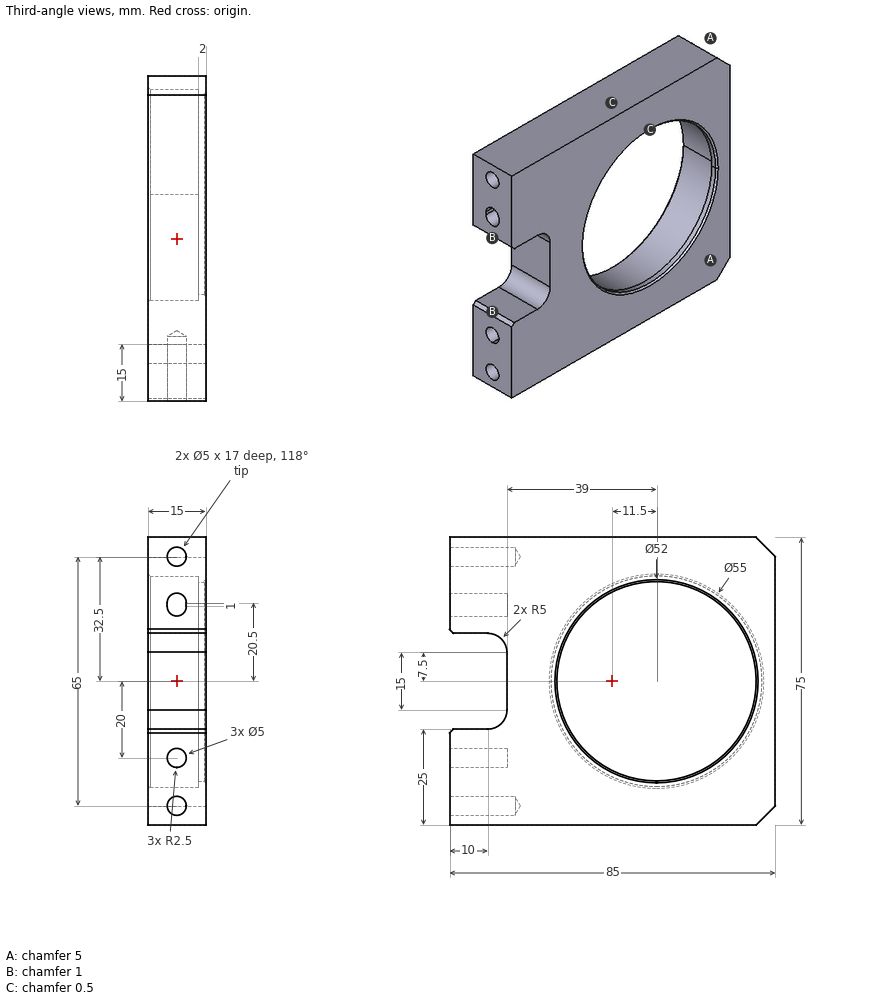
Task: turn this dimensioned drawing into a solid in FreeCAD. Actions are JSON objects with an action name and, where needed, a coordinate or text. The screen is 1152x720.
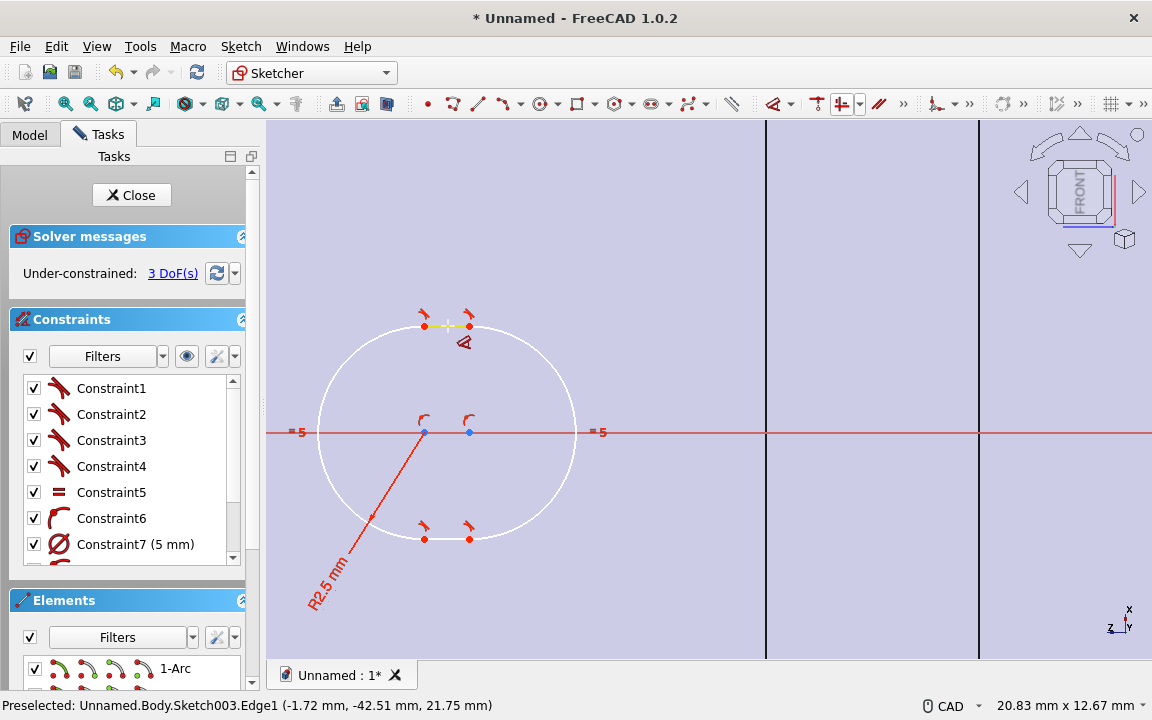
{"action": "left_click", "coordinate": [447, 327]}
{"action": "left_click", "coordinate": [447, 293]}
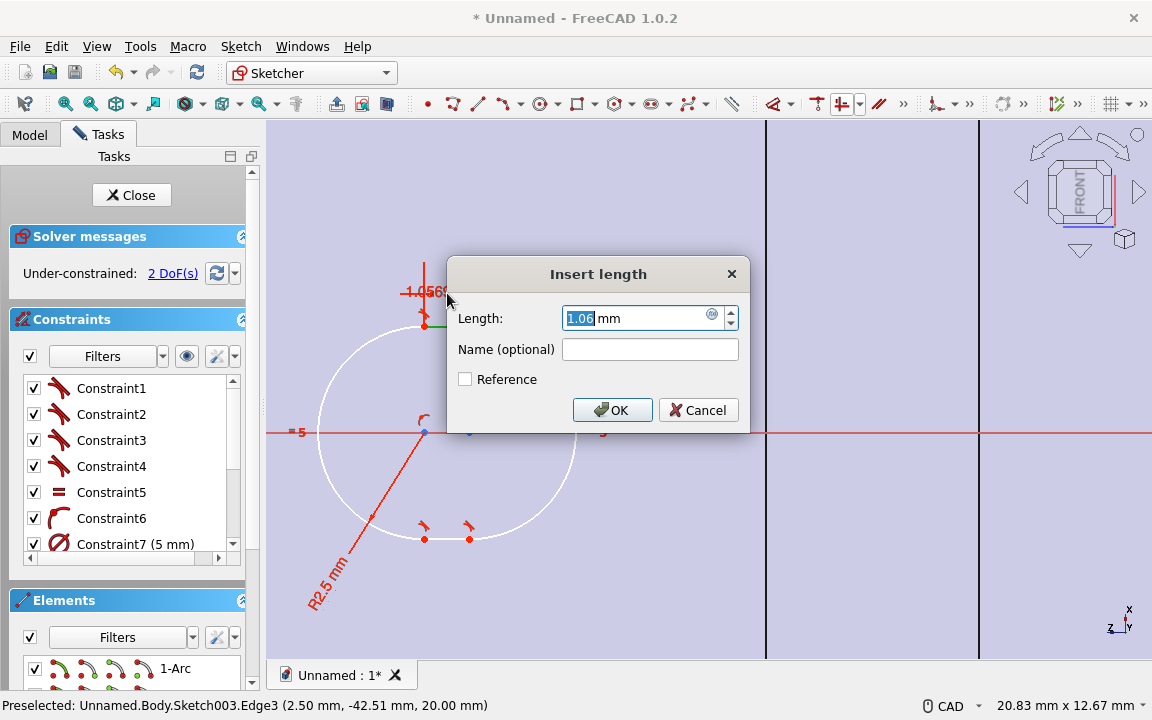
{"action": "type", "text": "1"}
{"action": "key", "text": "Return"}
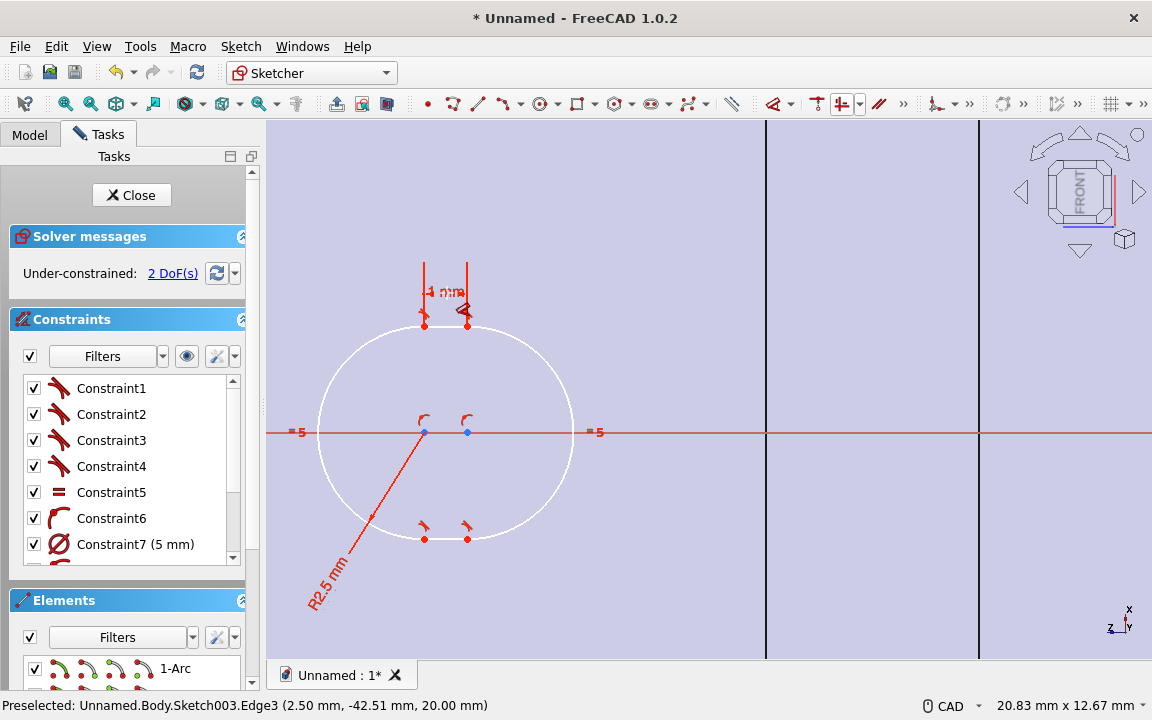
{"action": "scroll", "coordinate": [429, 375], "scroll_direction": "down", "scroll_amount": 7}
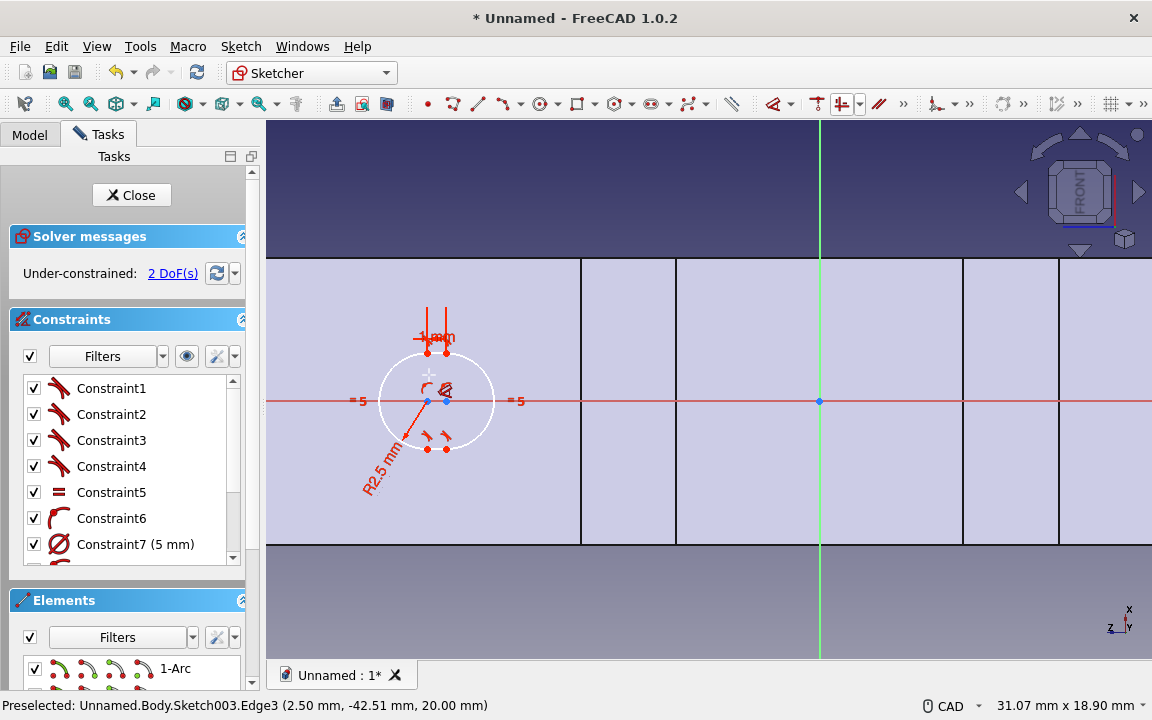
{"action": "left_click", "coordinate": [853, 390]}
{"action": "left_click", "coordinate": [748, 424]}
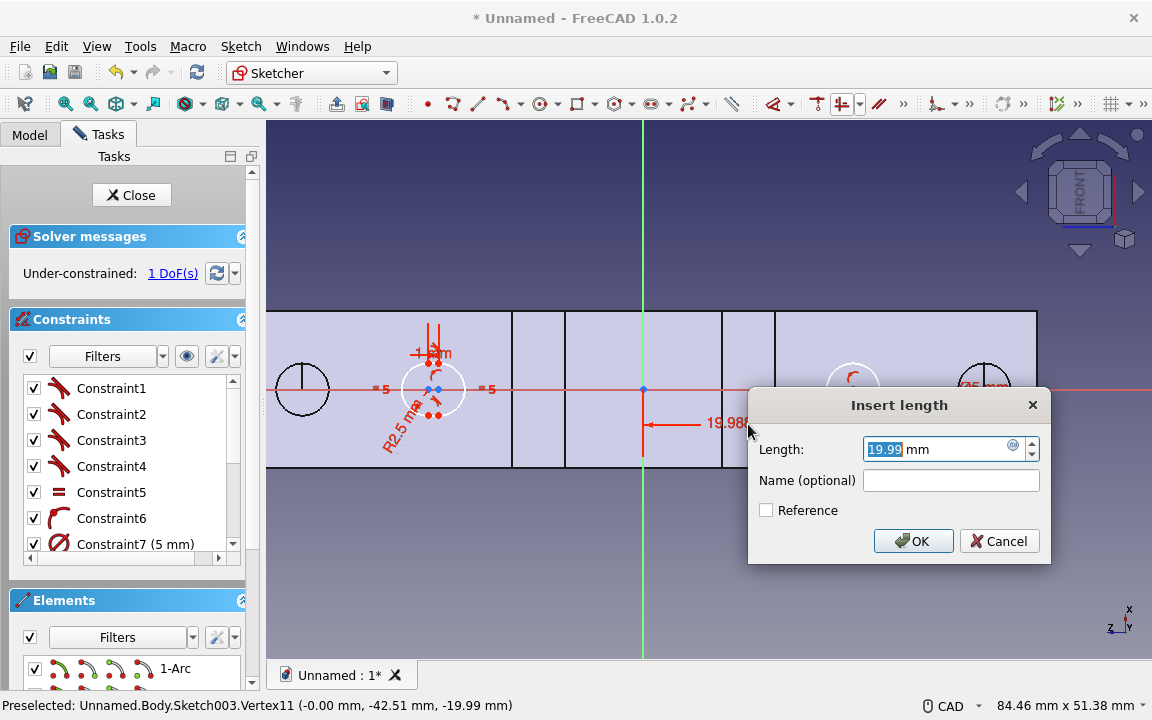
{"action": "type", "text": "20"}
{"action": "key", "text": "Return"}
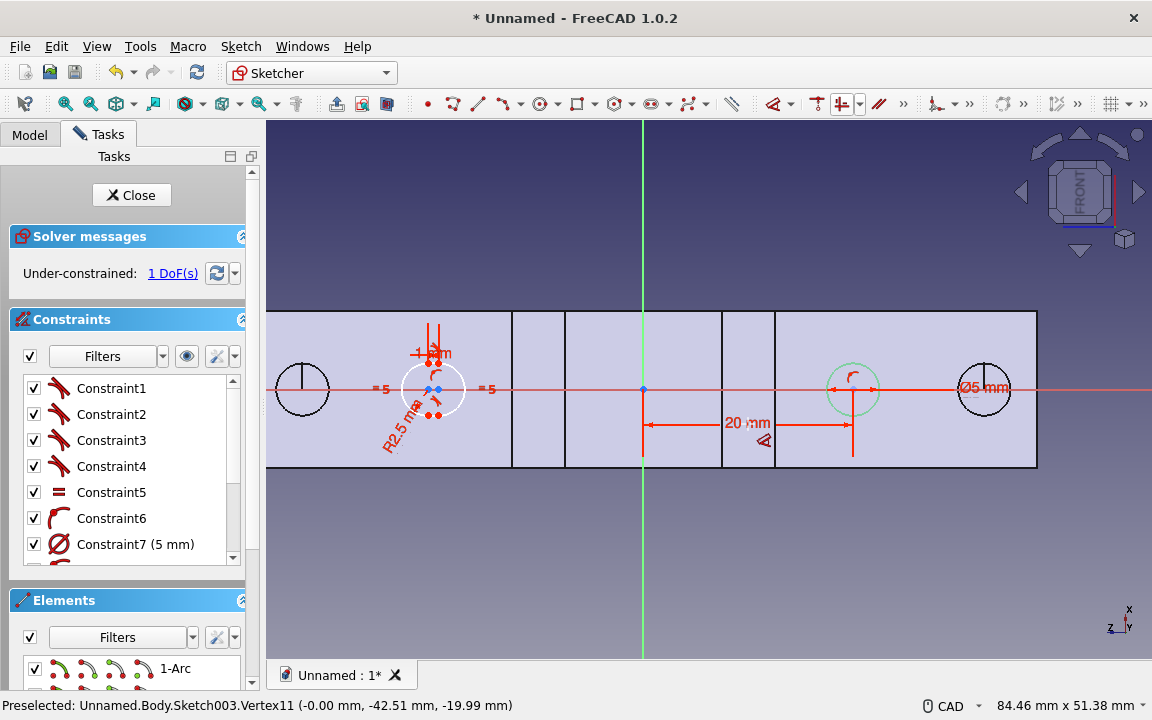
{"action": "left_click", "coordinate": [428, 363]}
{"action": "left_click", "coordinate": [536, 329]}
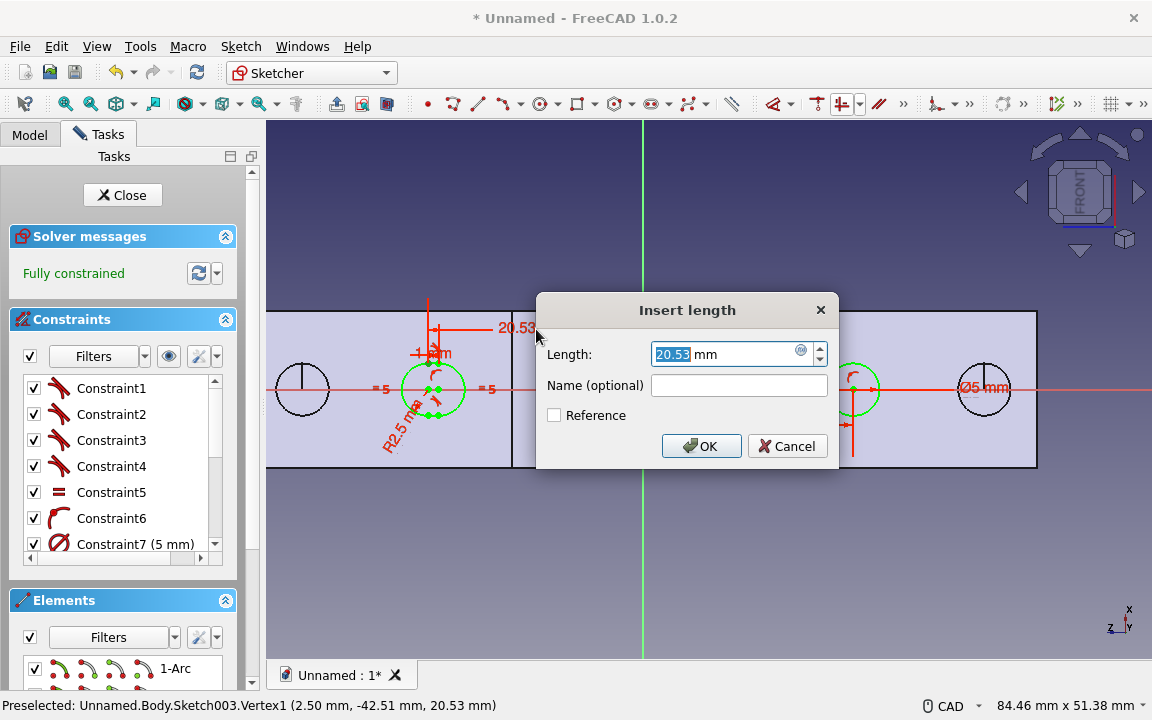
{"action": "type", "text": "20.5"}
{"action": "key", "text": "Return"}
{"action": "key", "text": "Escape"}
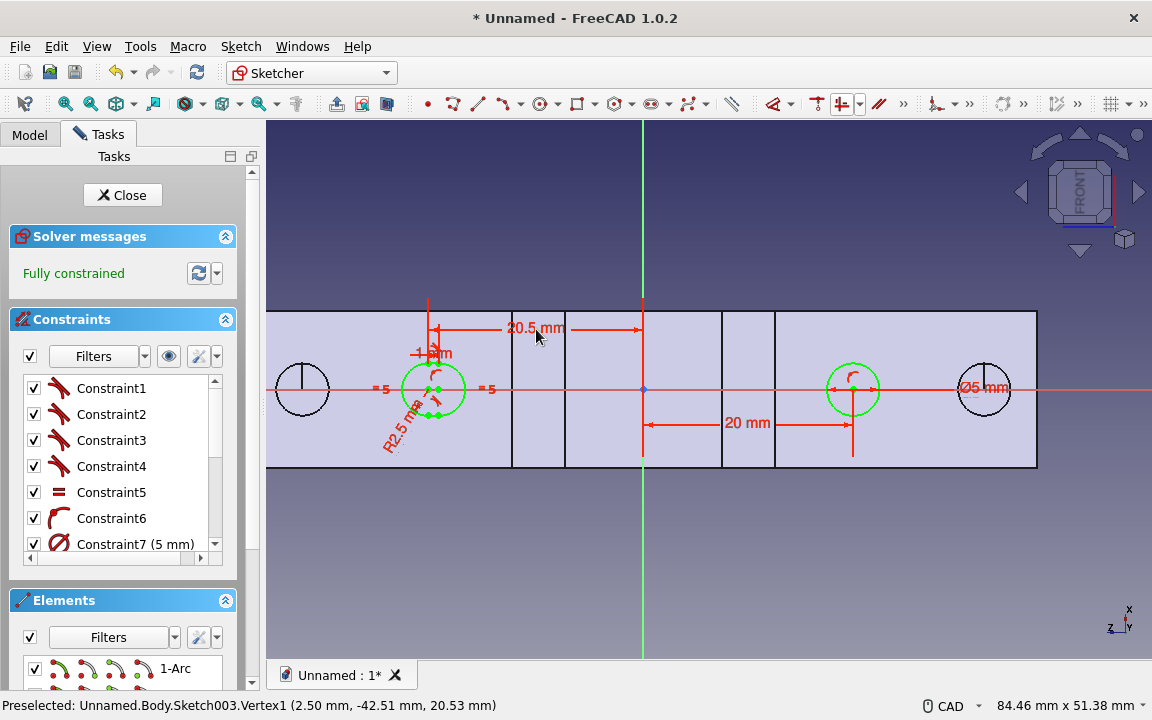
{"action": "left_click", "coordinate": [123, 195]}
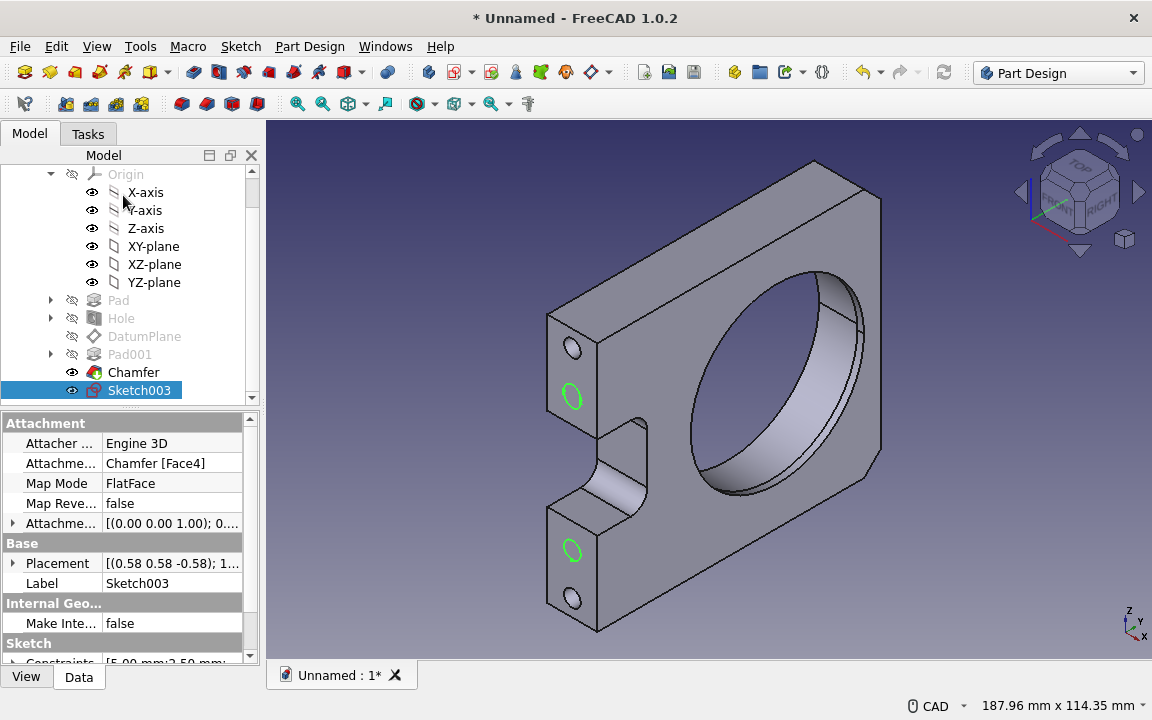
{"action": "left_click", "coordinate": [194, 72]}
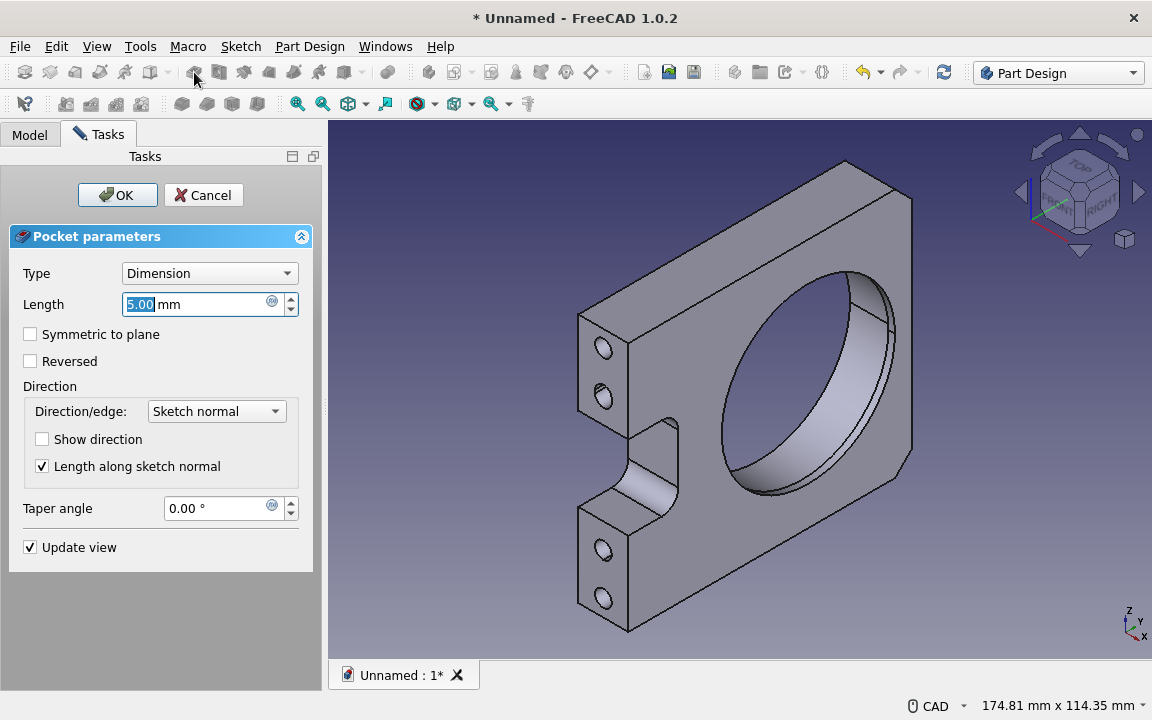
{"action": "type", "text": "15"}
{"action": "key", "text": "Tab"}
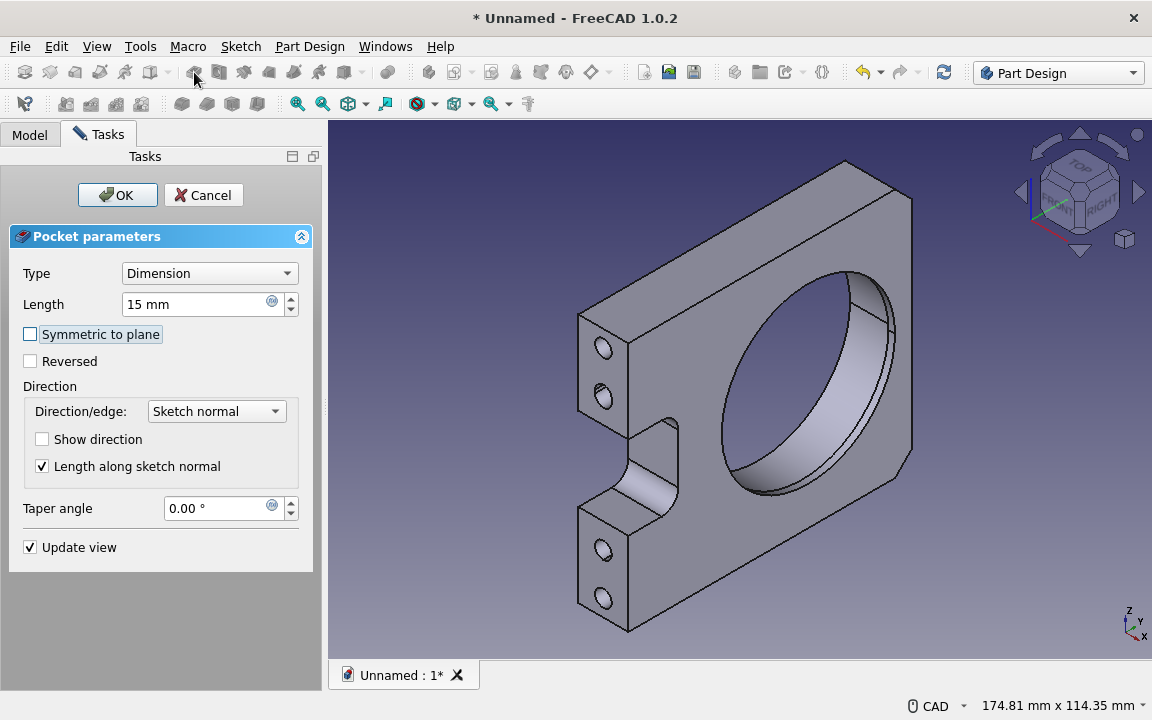
{"action": "left_click", "coordinate": [118, 195]}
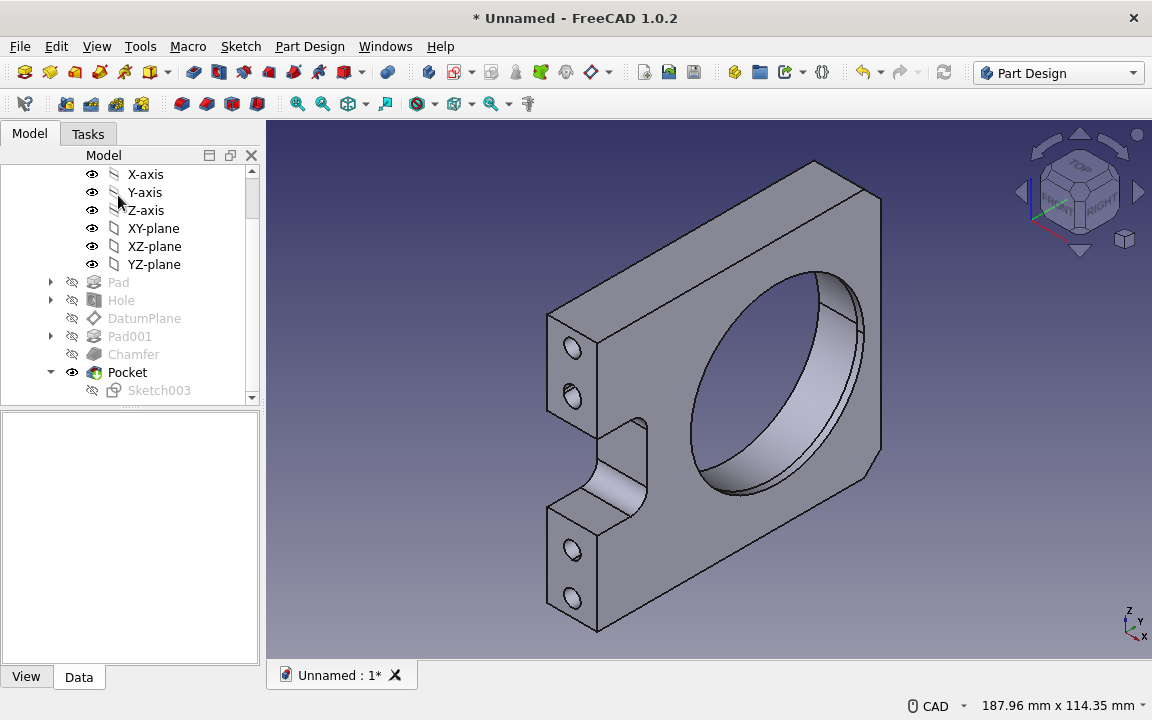
{"action": "left_click", "coordinate": [572, 520]}